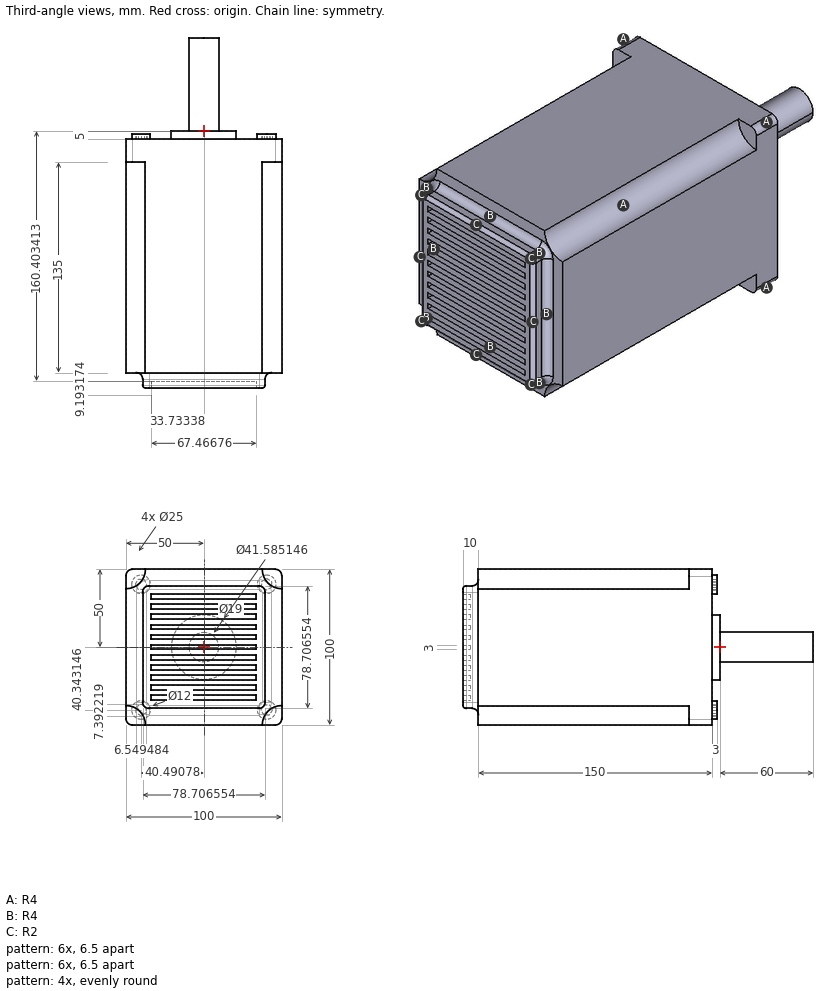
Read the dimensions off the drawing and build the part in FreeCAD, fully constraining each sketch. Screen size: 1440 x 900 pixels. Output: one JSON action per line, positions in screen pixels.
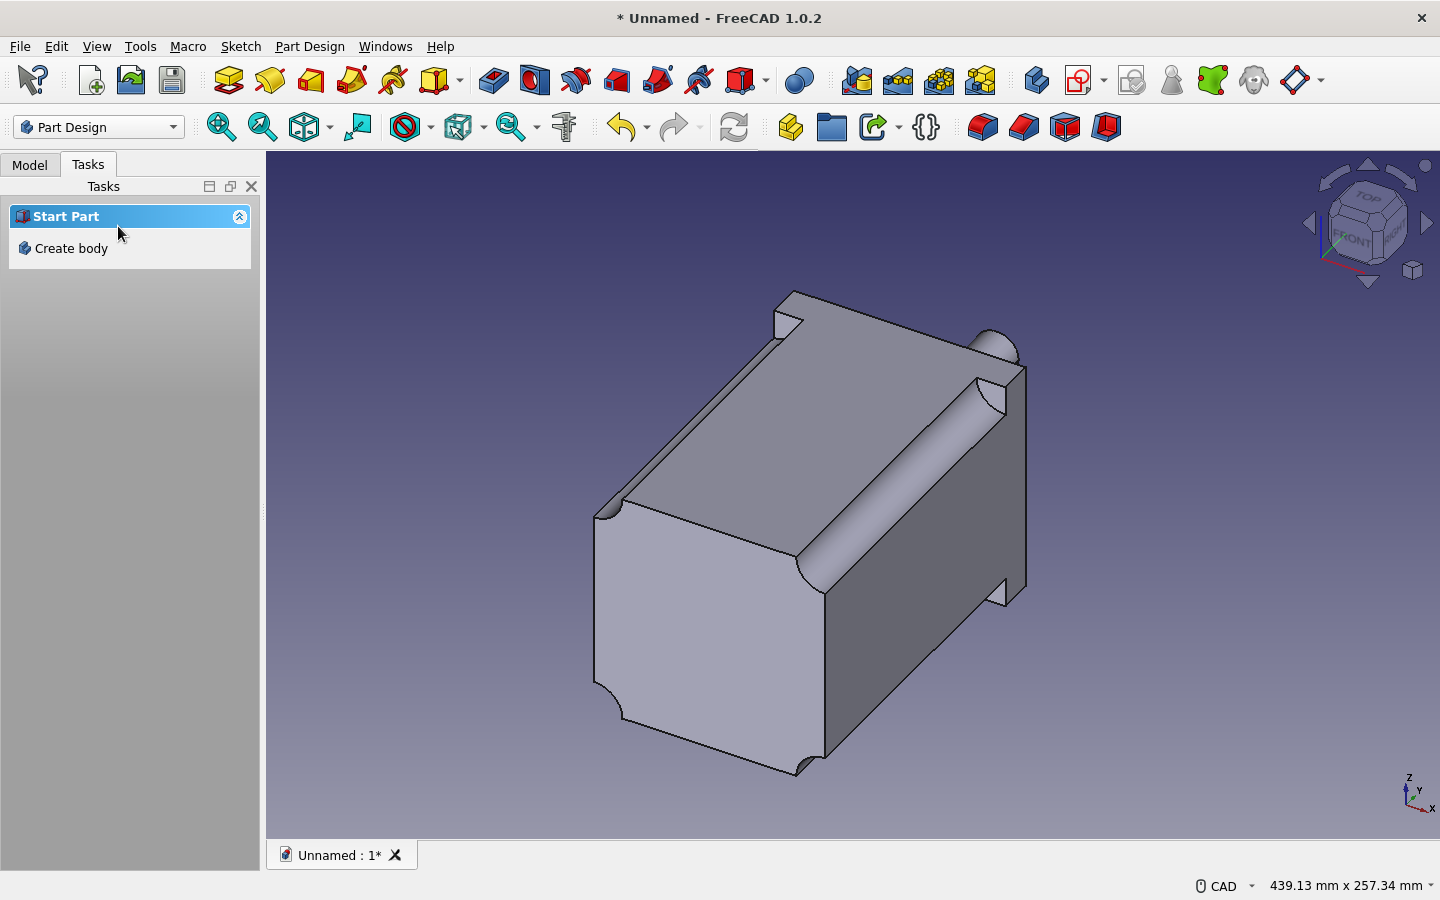
{"action": "left_click", "coordinate": [1016, 376]}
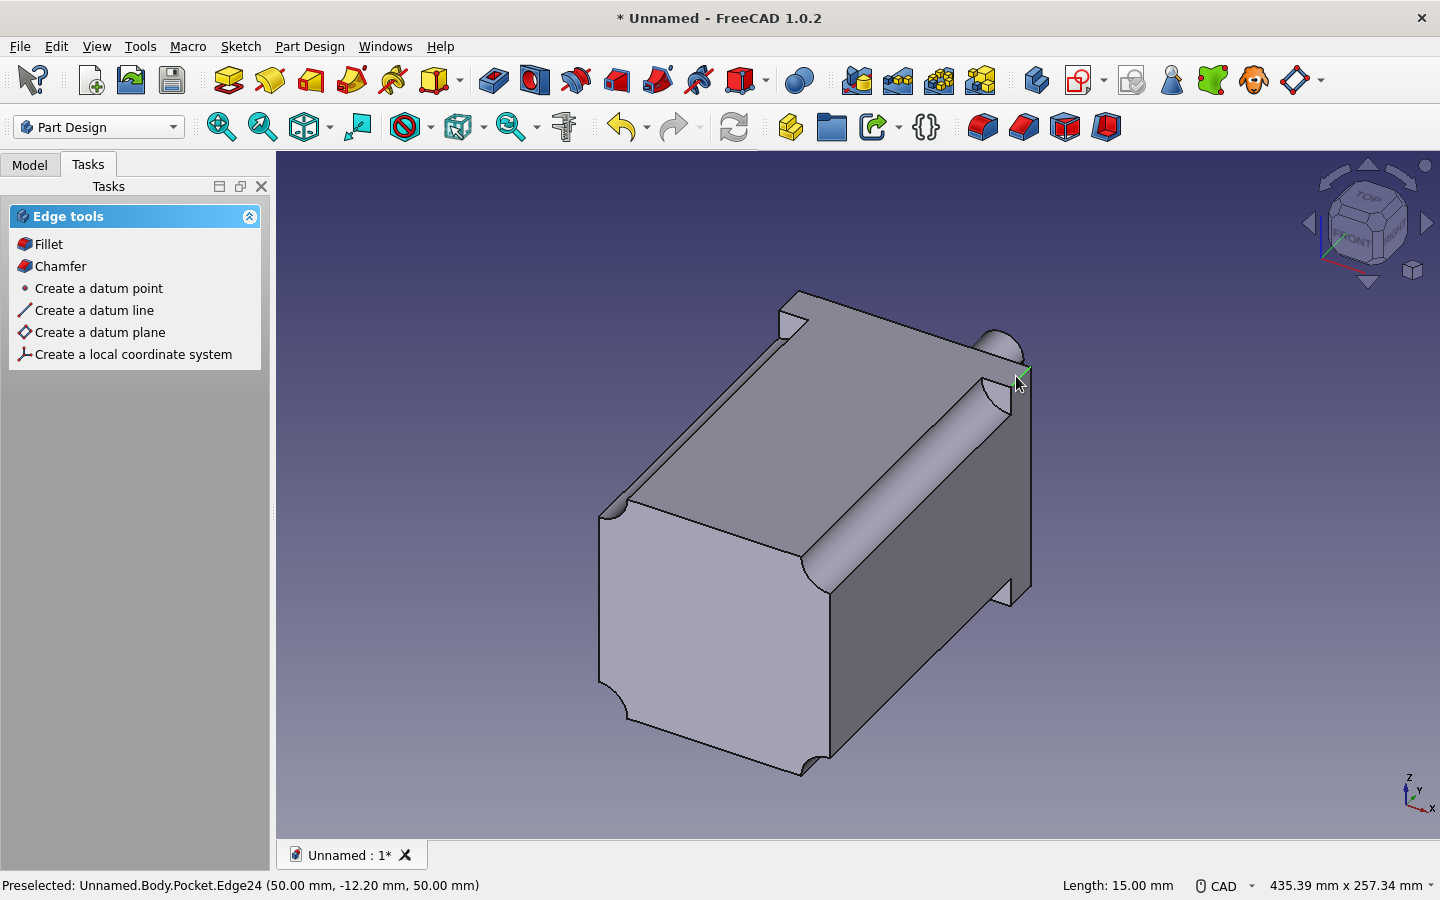
{"action": "key", "text": "0"}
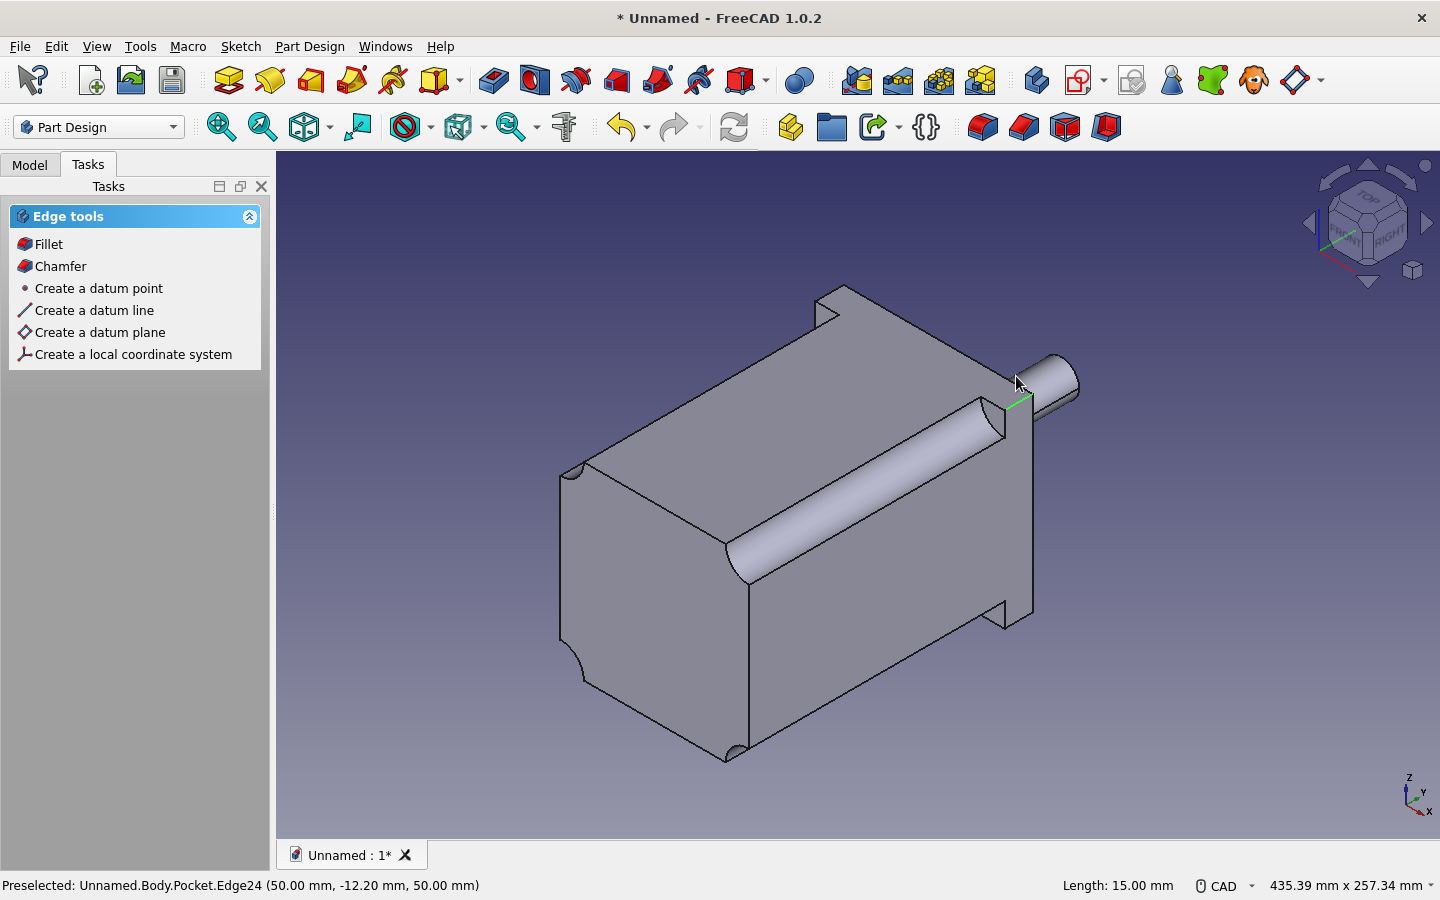
{"action": "key", "text": "2"}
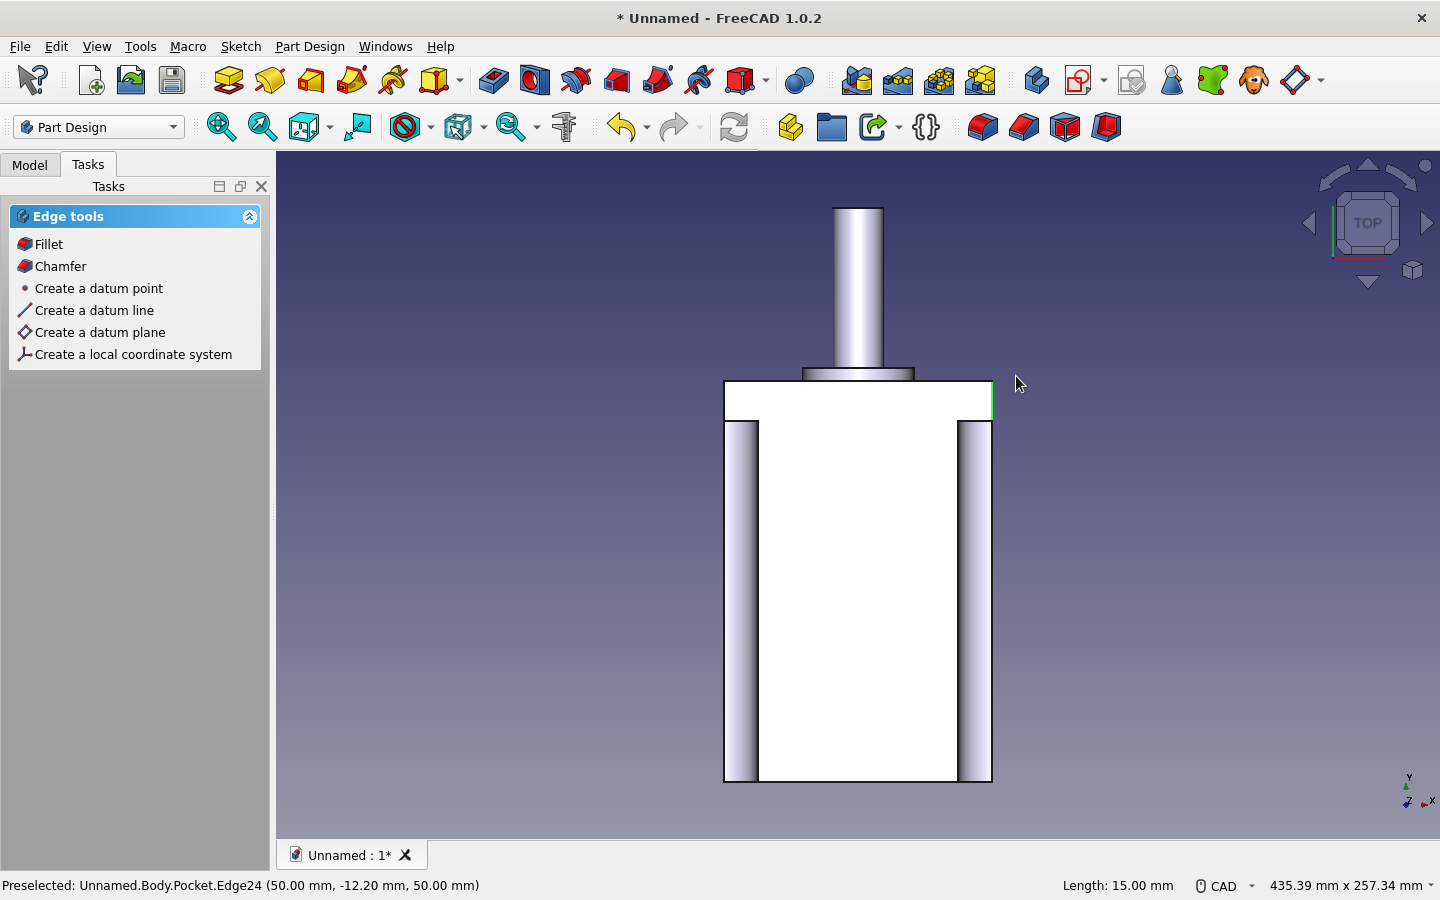
{"action": "left_click", "coordinate": [724, 400], "text": "ctrl"}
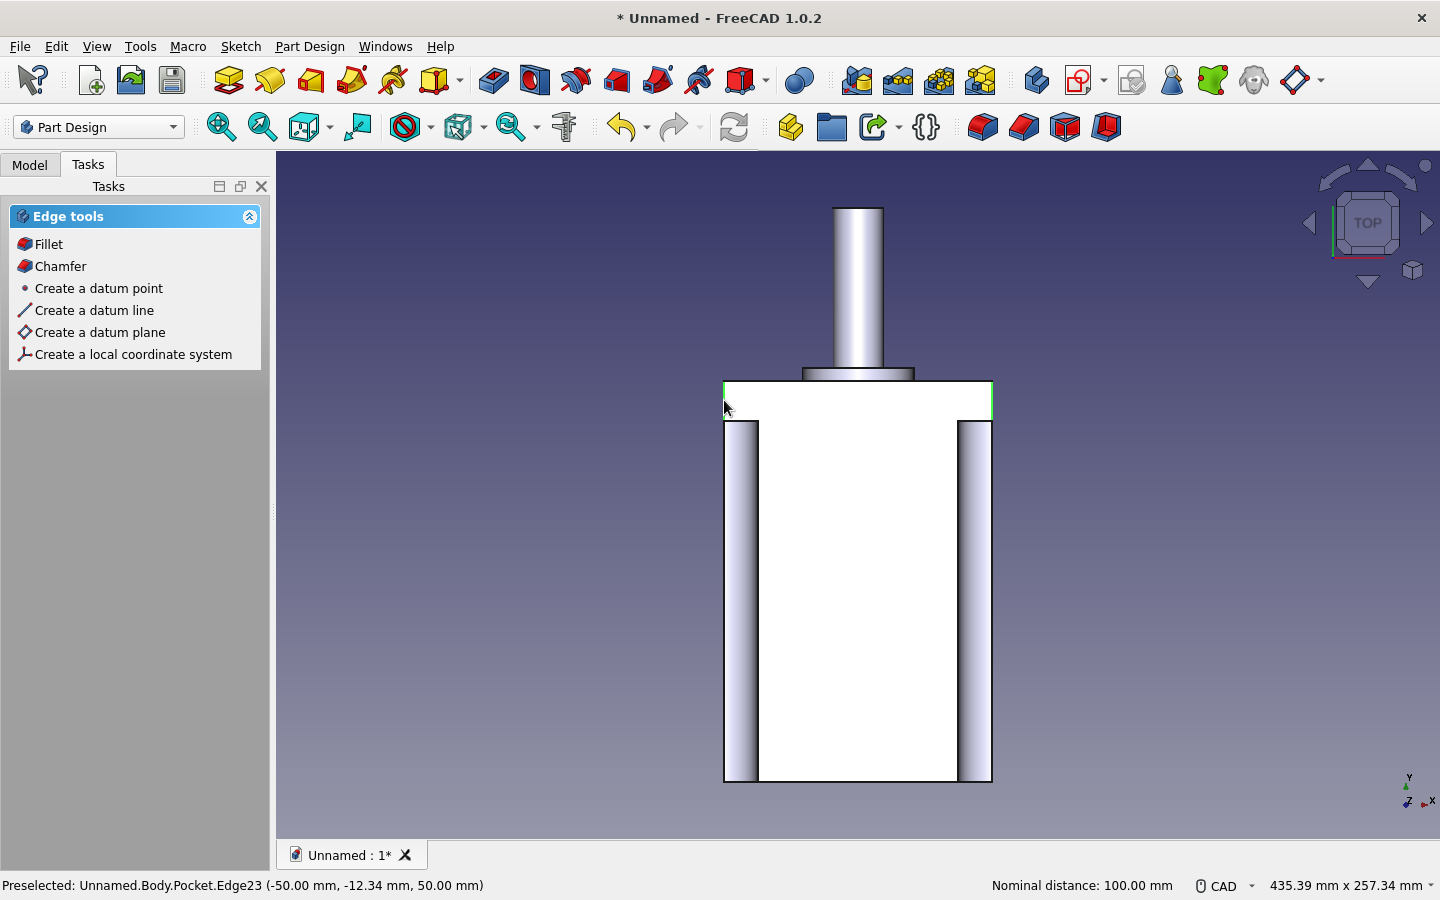
{"action": "key", "text": "1"}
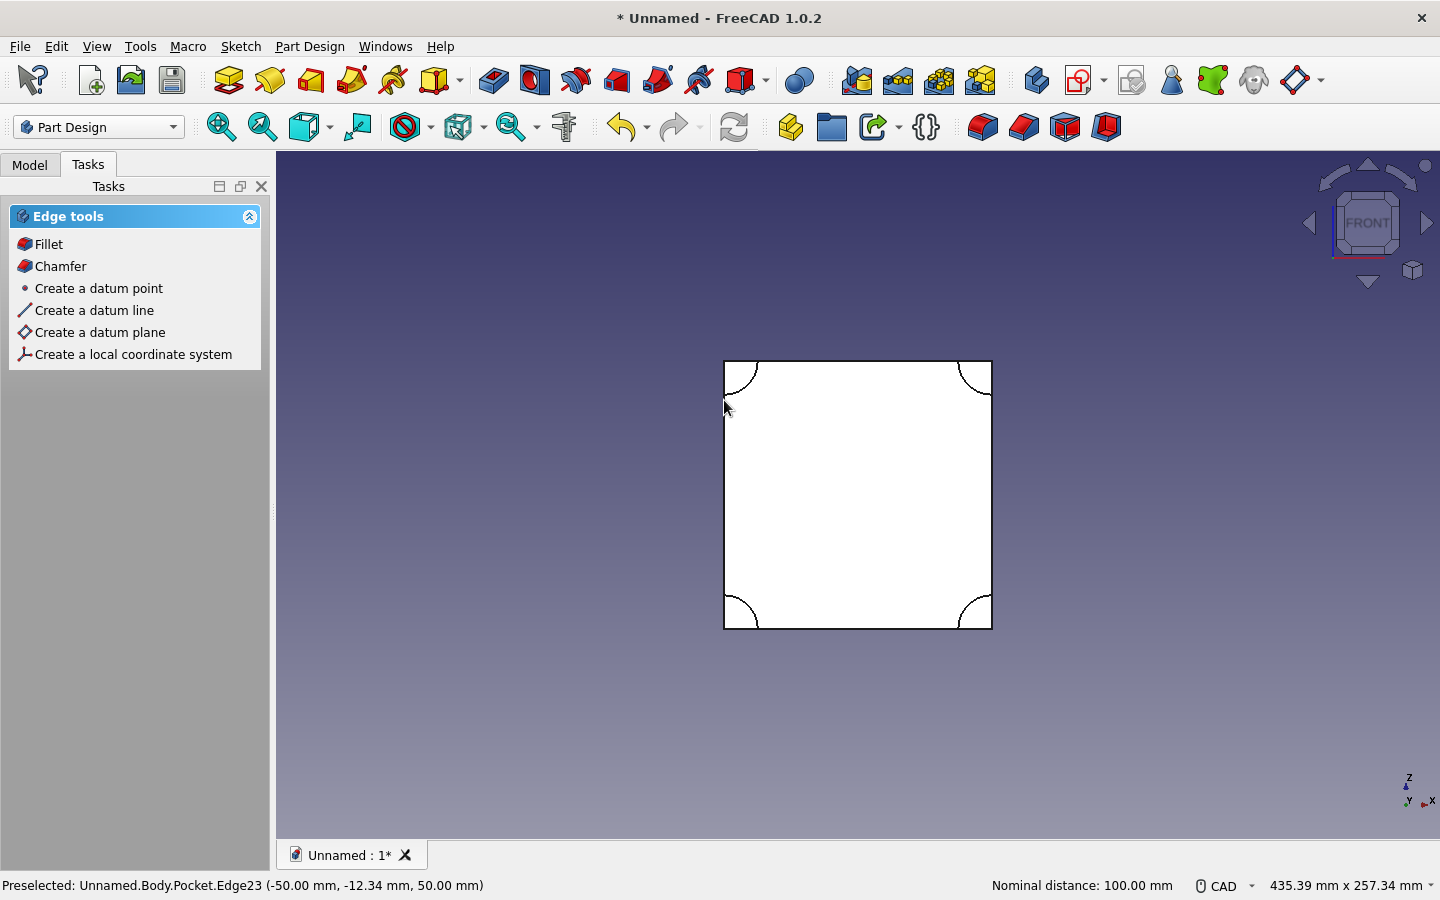
{"action": "key", "text": "v f"}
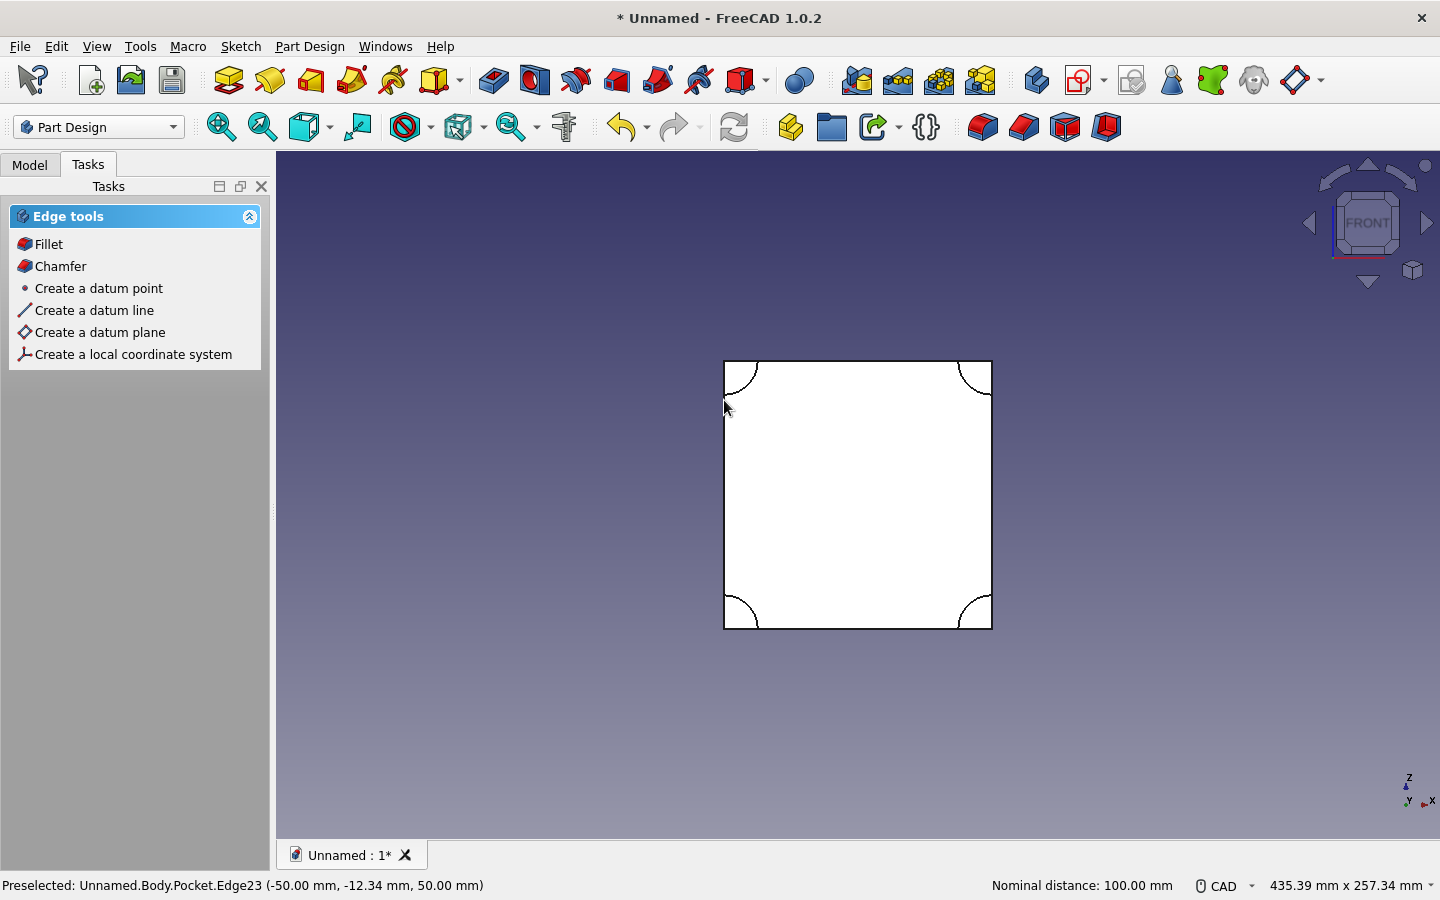
{"action": "key", "text": "3"}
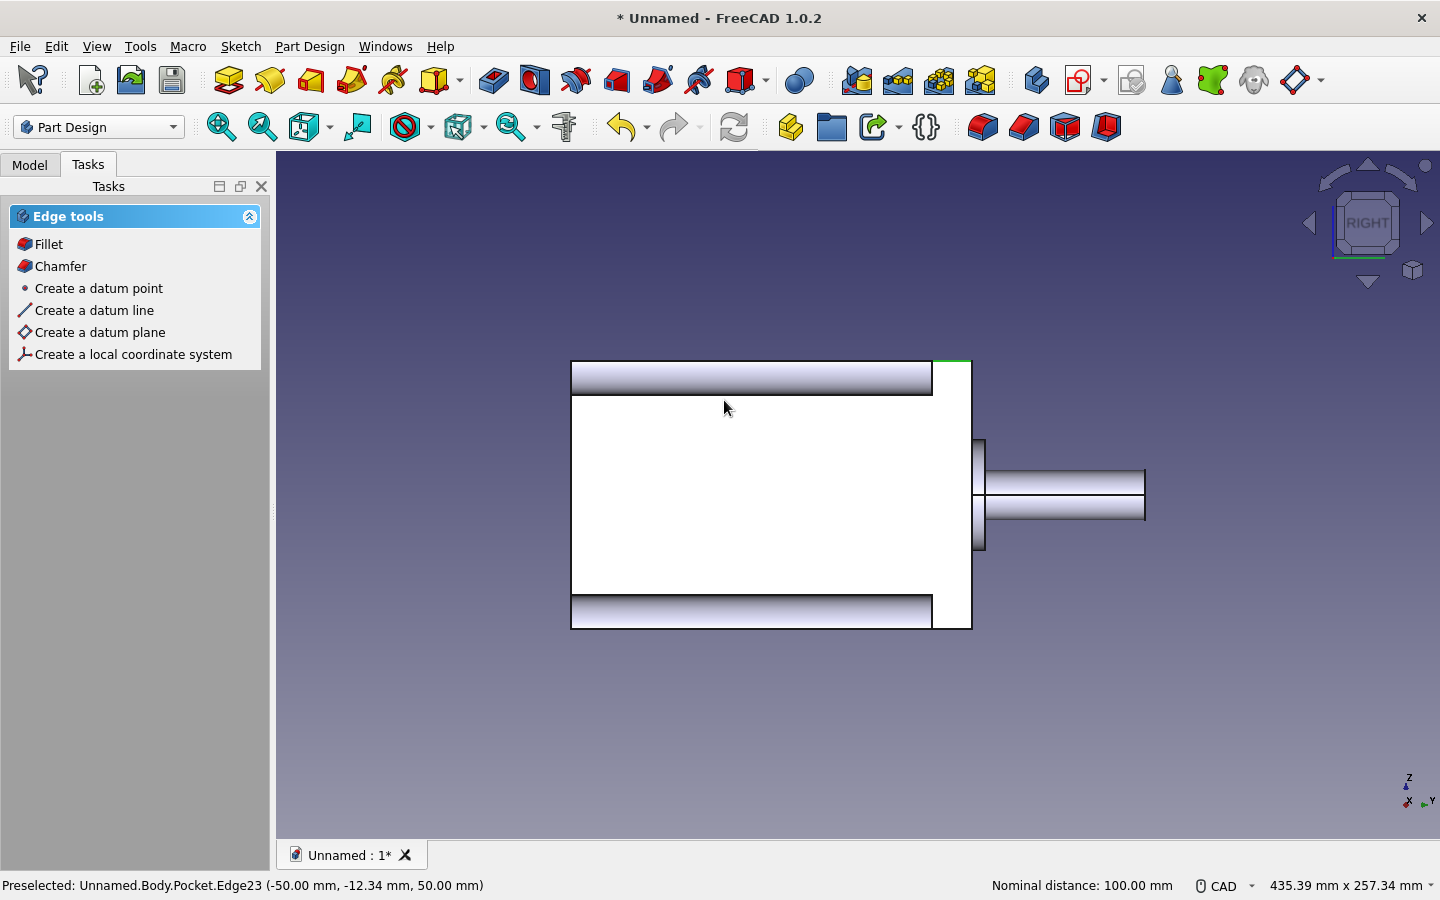
{"action": "left_click", "coordinate": [952, 628], "text": "ctrl"}